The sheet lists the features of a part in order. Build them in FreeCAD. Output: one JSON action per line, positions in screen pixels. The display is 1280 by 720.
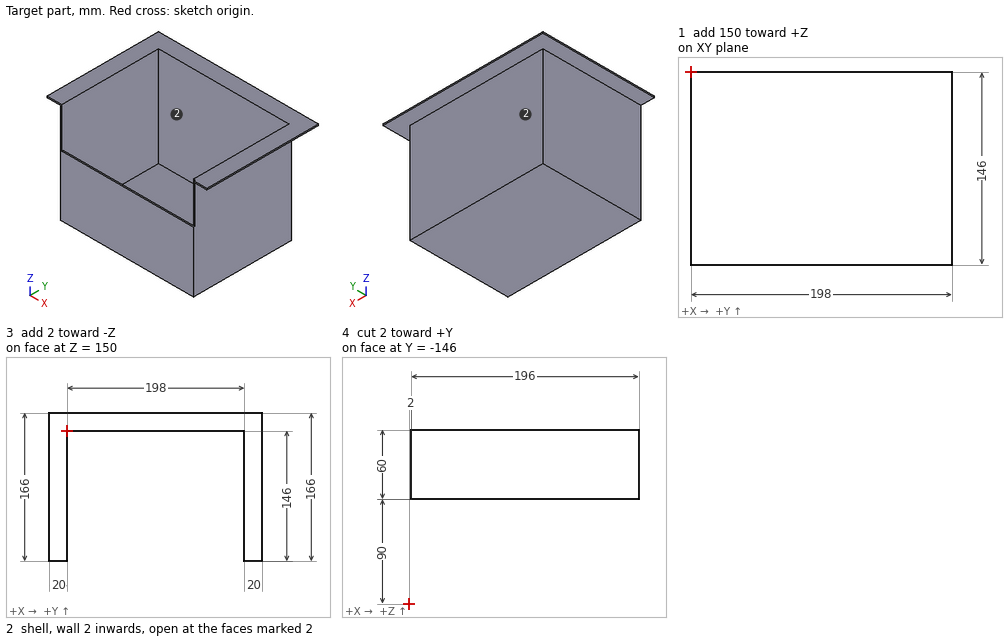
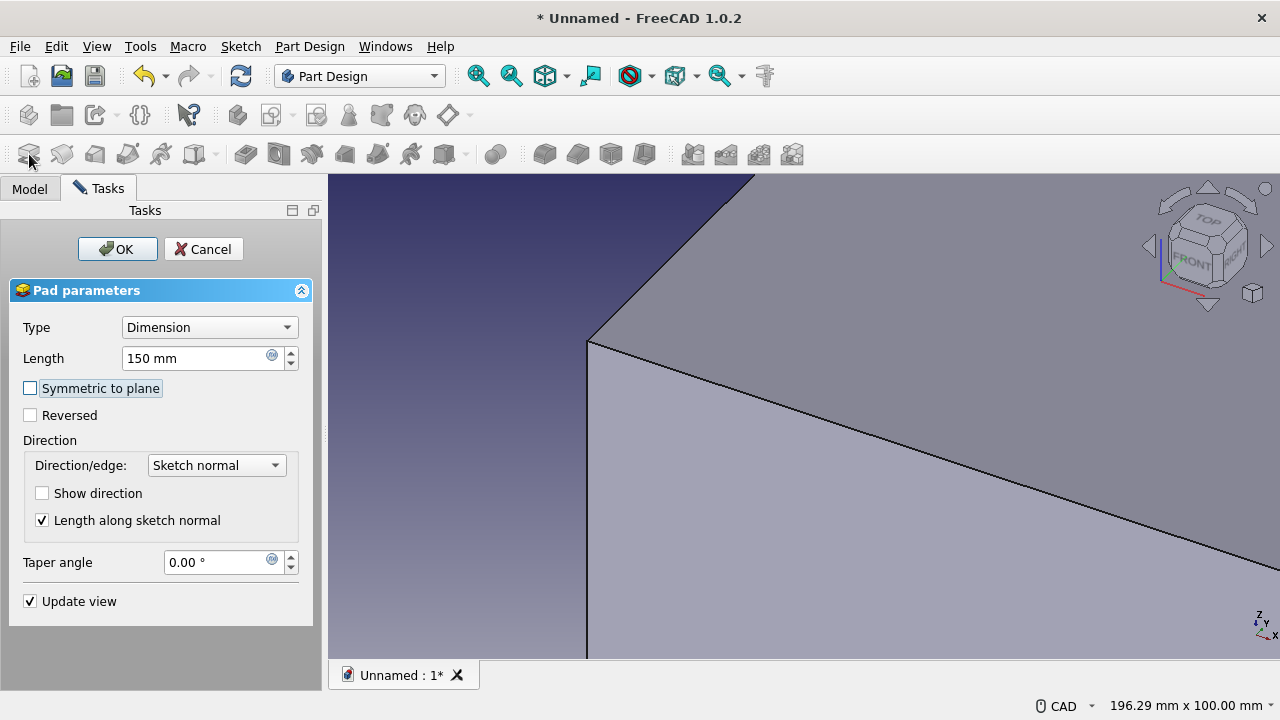
{"action": "left_click", "coordinate": [118, 249]}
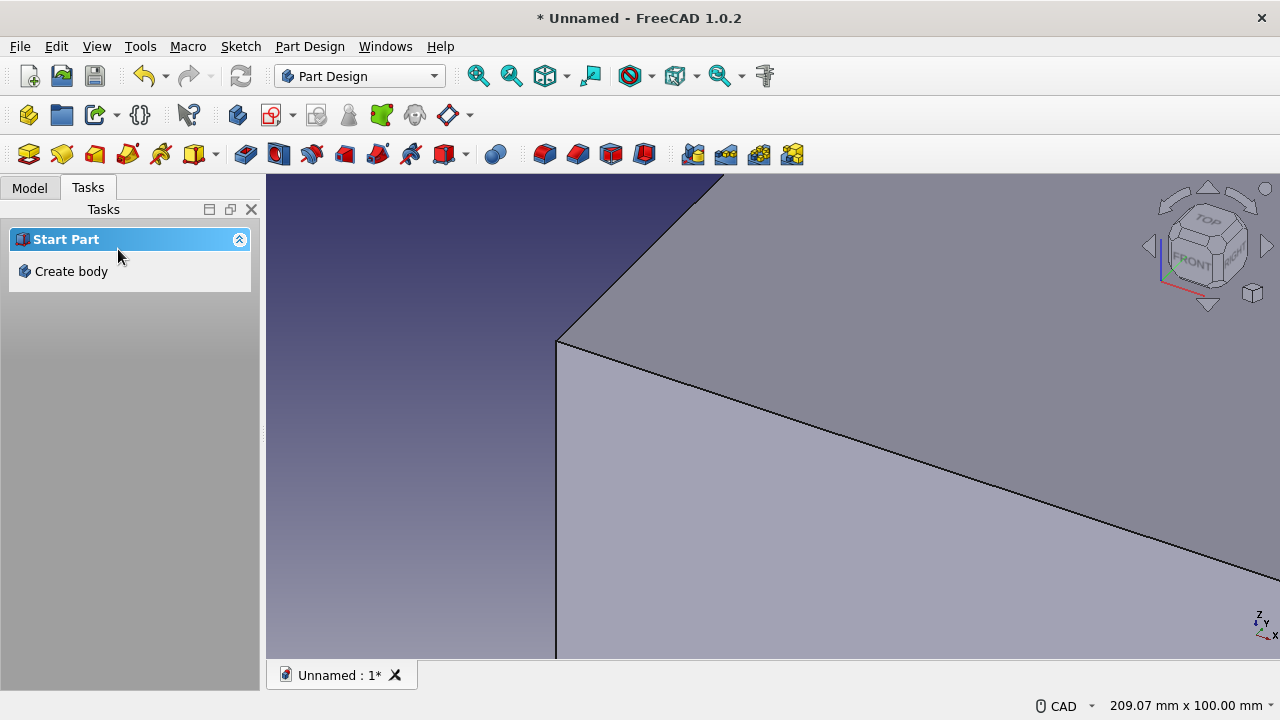
{"action": "left_click", "coordinate": [479, 76]}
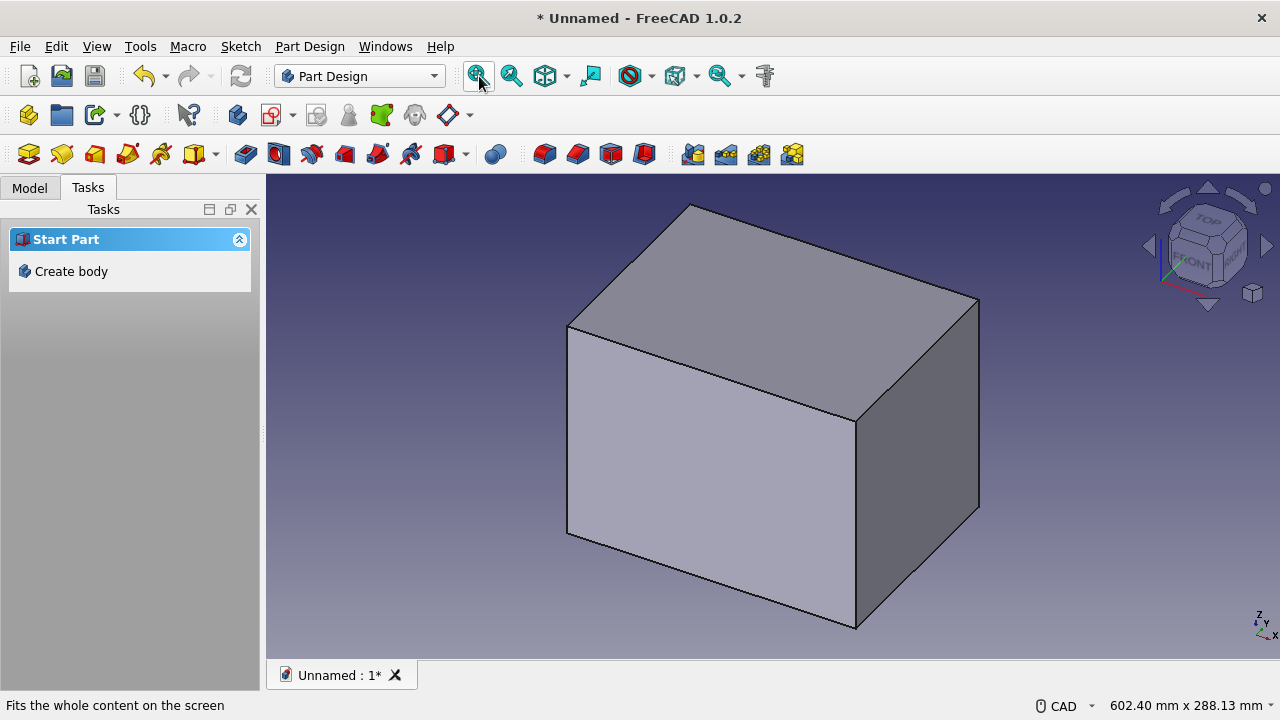
{"action": "left_click", "coordinate": [773, 312]}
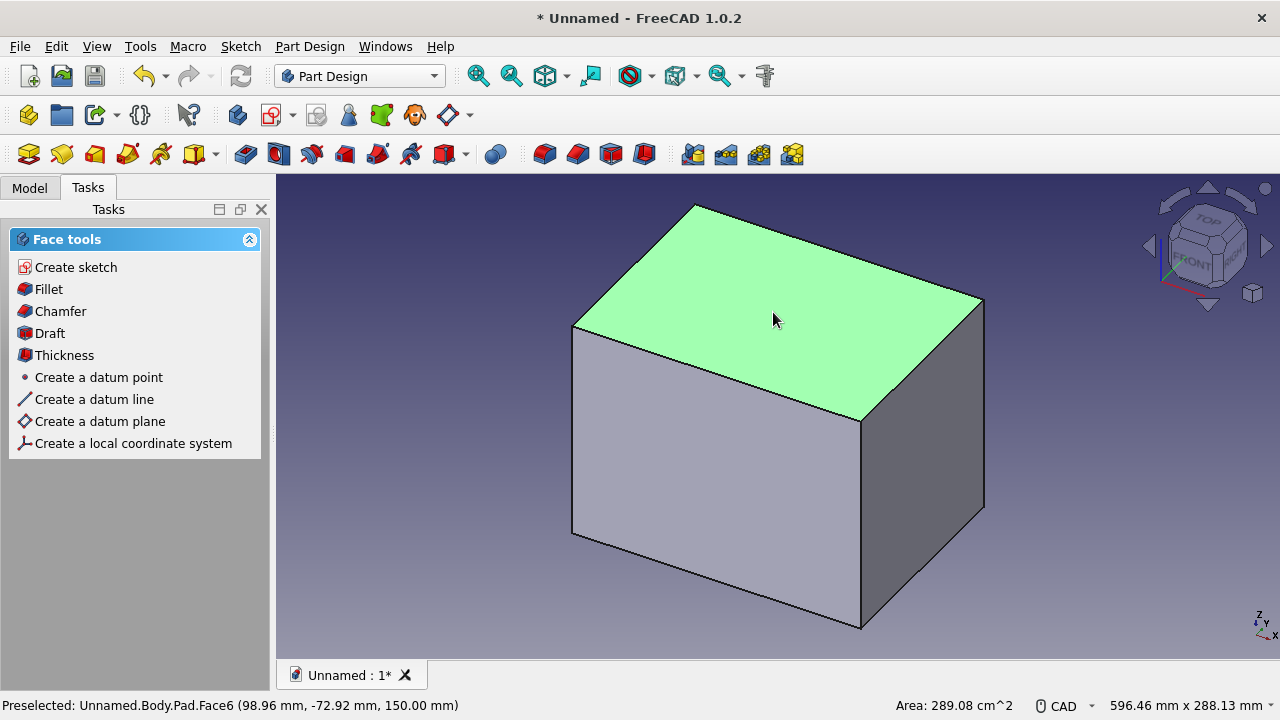
{"action": "left_click", "coordinate": [644, 154]}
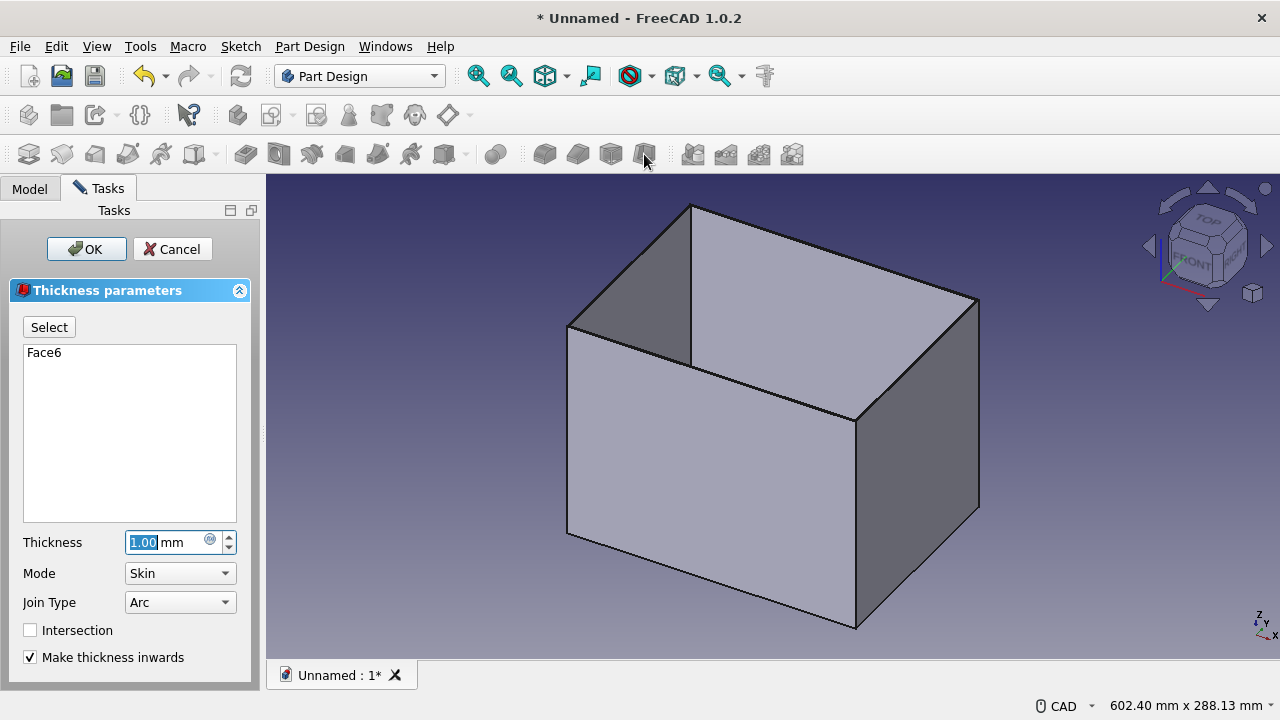
{"action": "type", "text": "2"}
{"action": "key", "text": "Tab"}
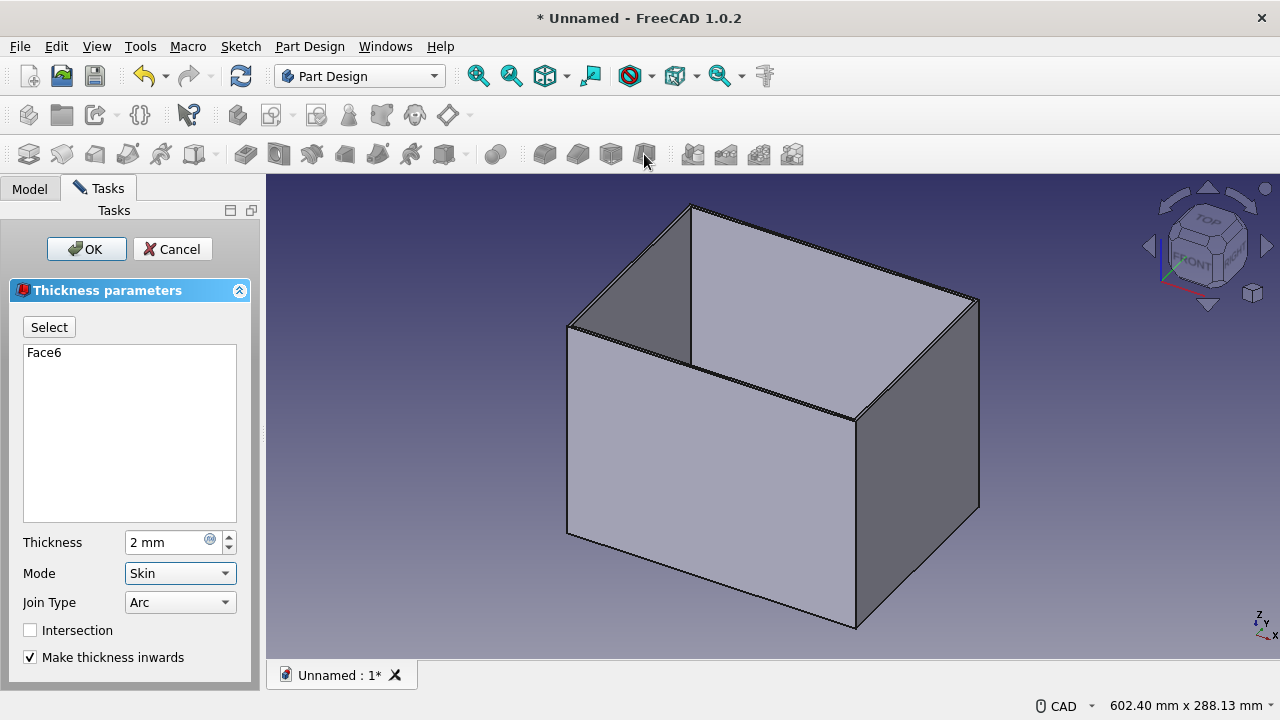
{"action": "left_click", "coordinate": [181, 602]}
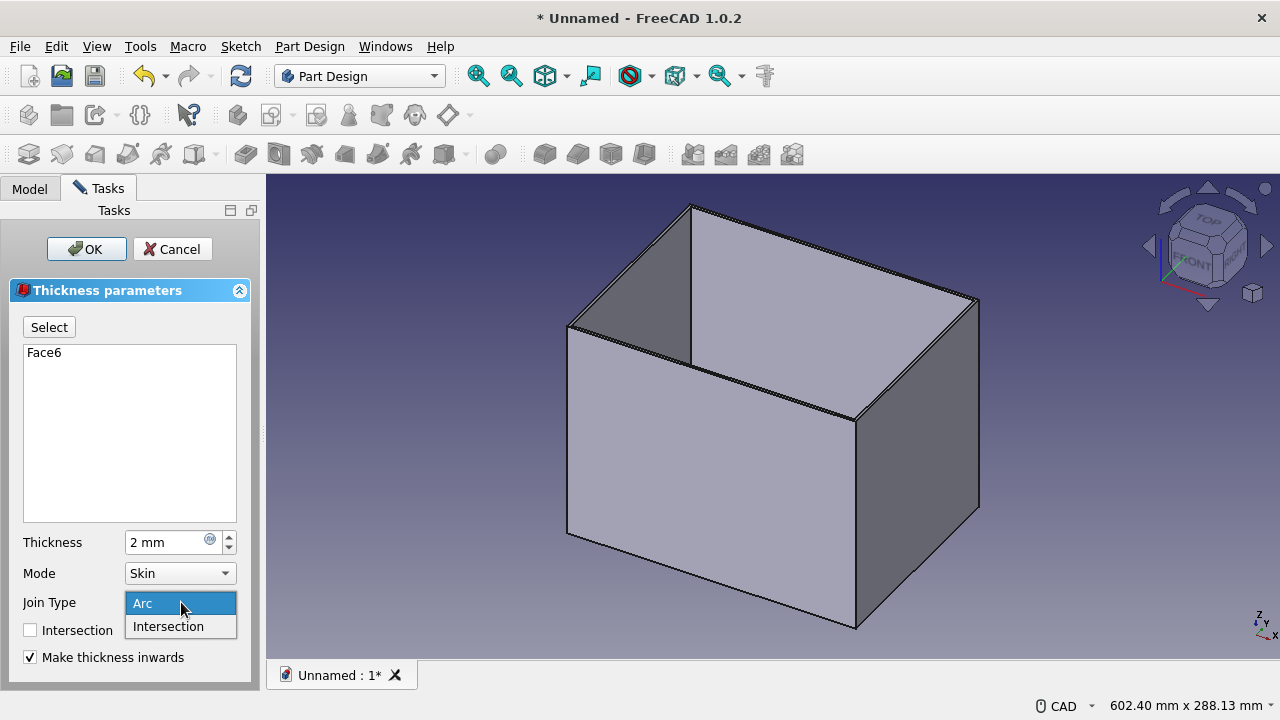
{"action": "left_click", "coordinate": [179, 626]}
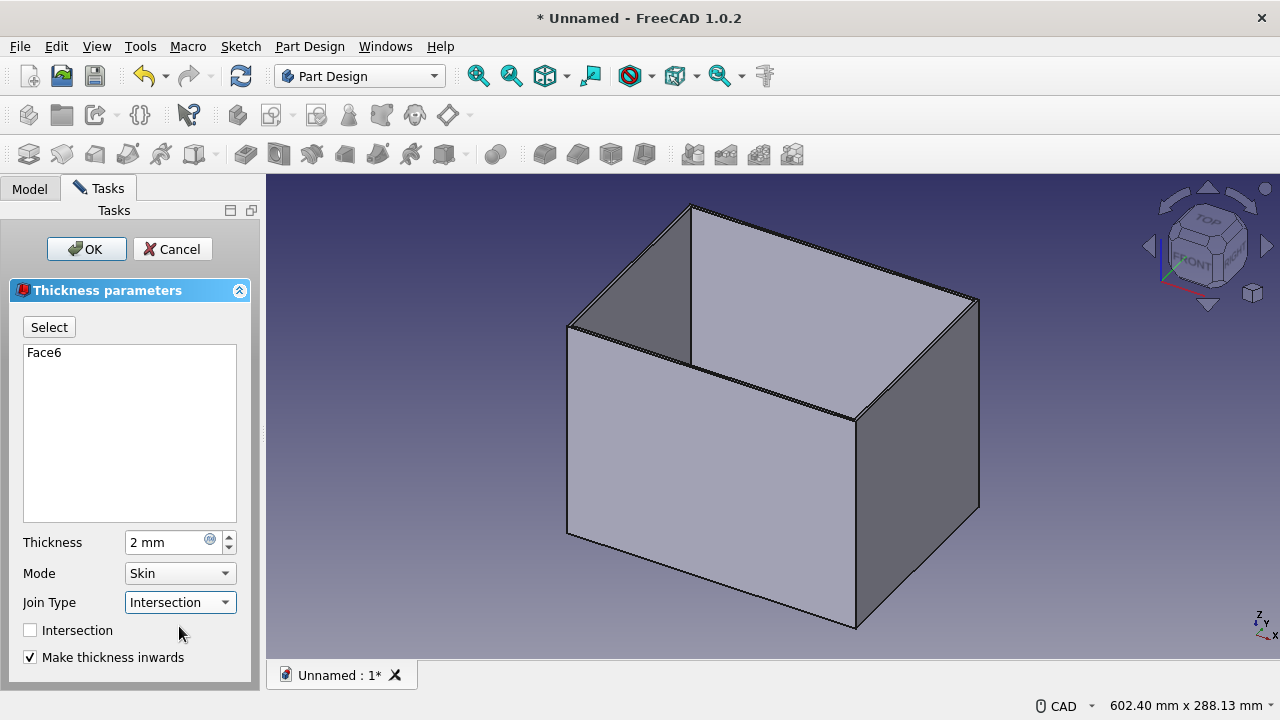
{"action": "left_click", "coordinate": [87, 249]}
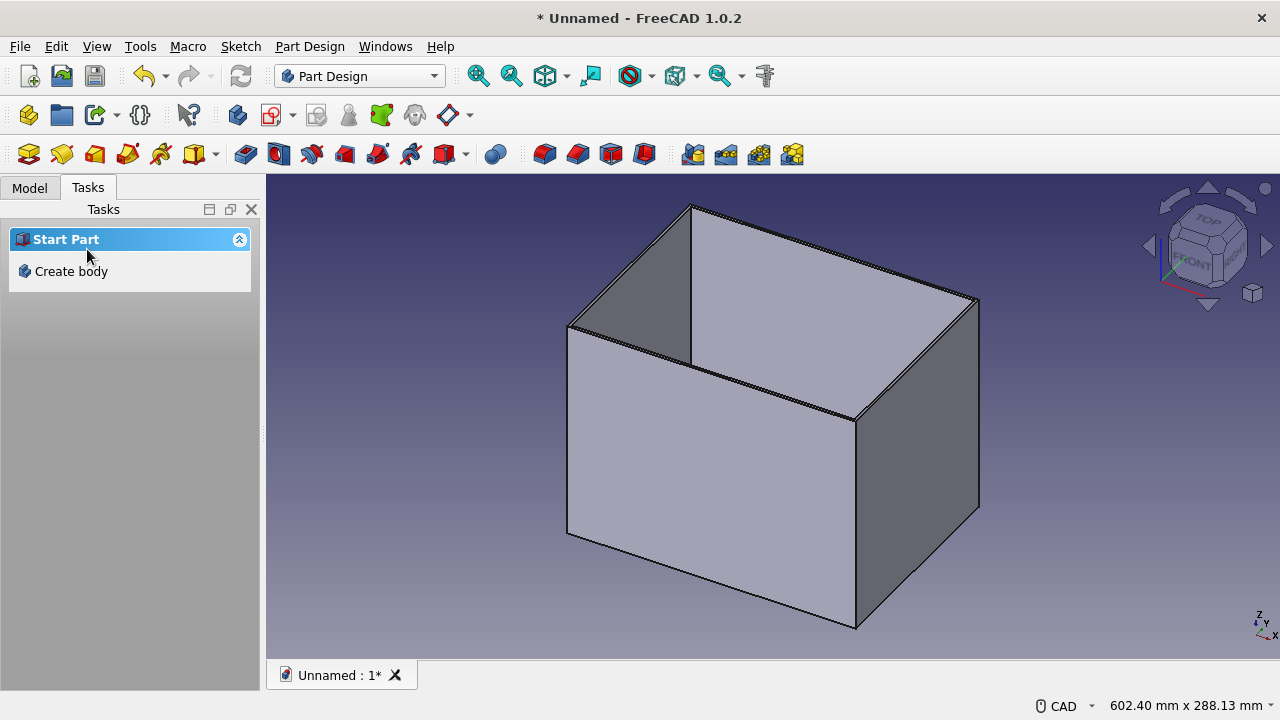
{"action": "scroll", "coordinate": [881, 268], "scroll_direction": "up", "scroll_amount": 12}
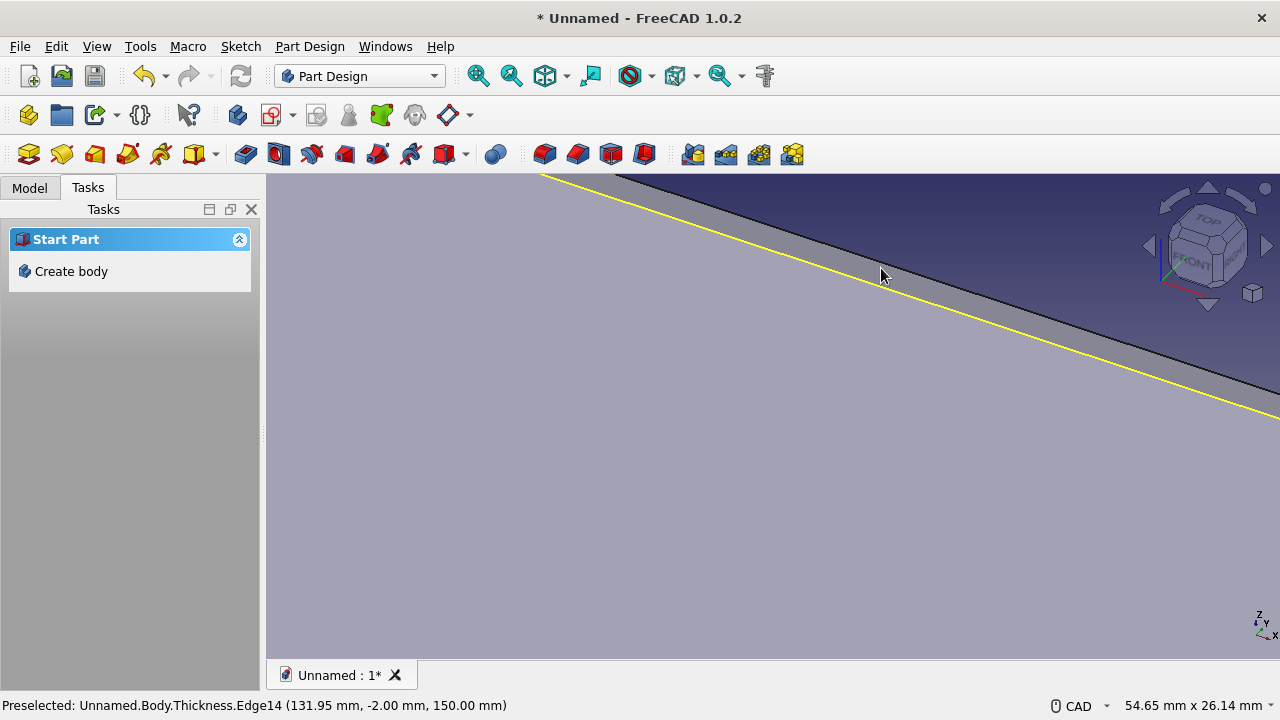
{"action": "left_click", "coordinate": [479, 76]}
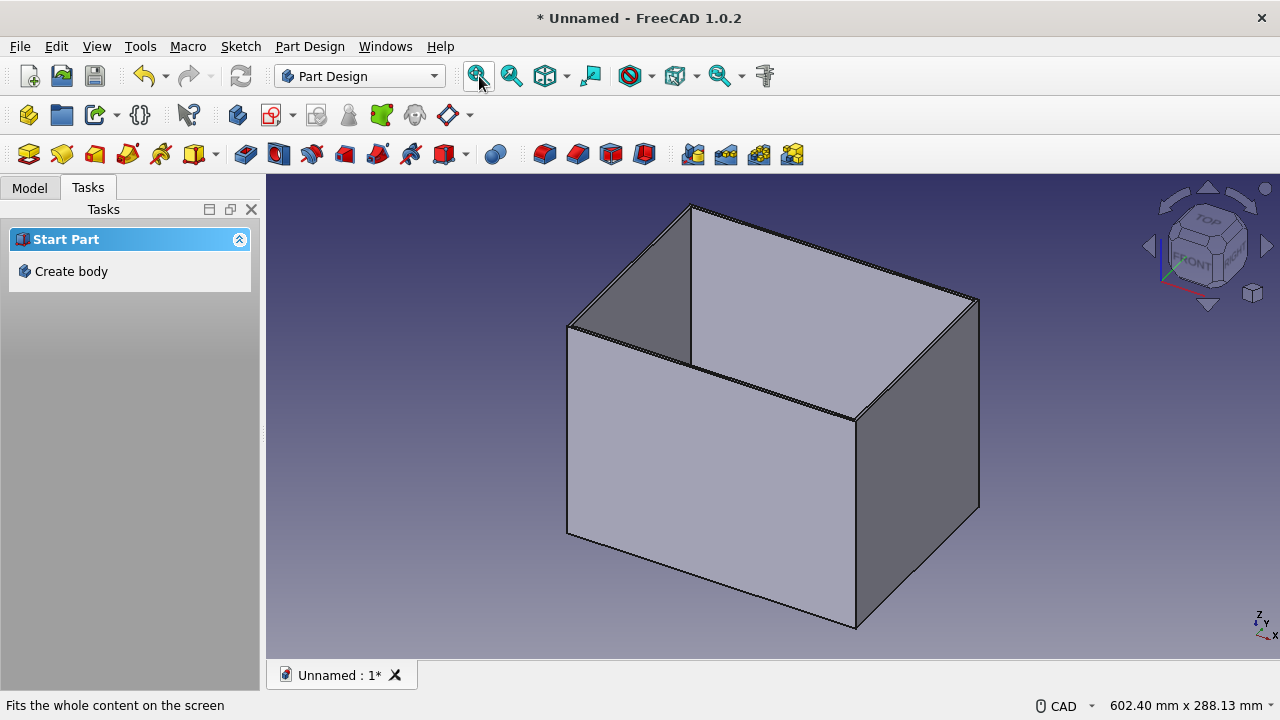
{"action": "key", "text": "0"}